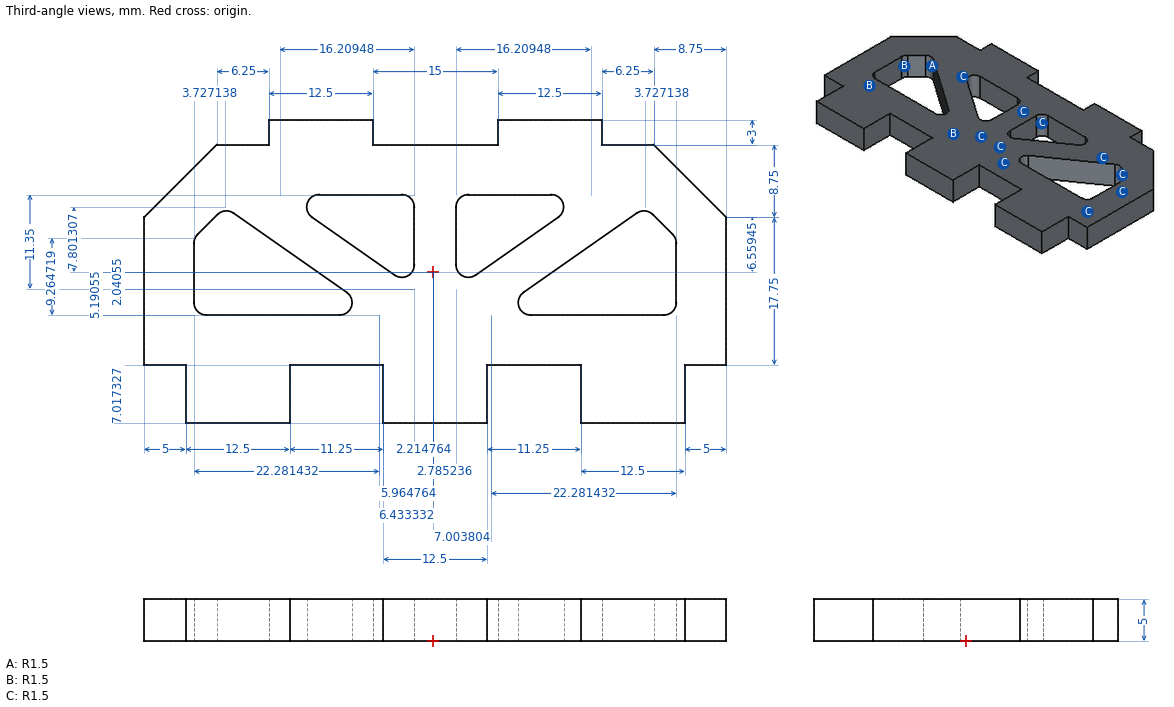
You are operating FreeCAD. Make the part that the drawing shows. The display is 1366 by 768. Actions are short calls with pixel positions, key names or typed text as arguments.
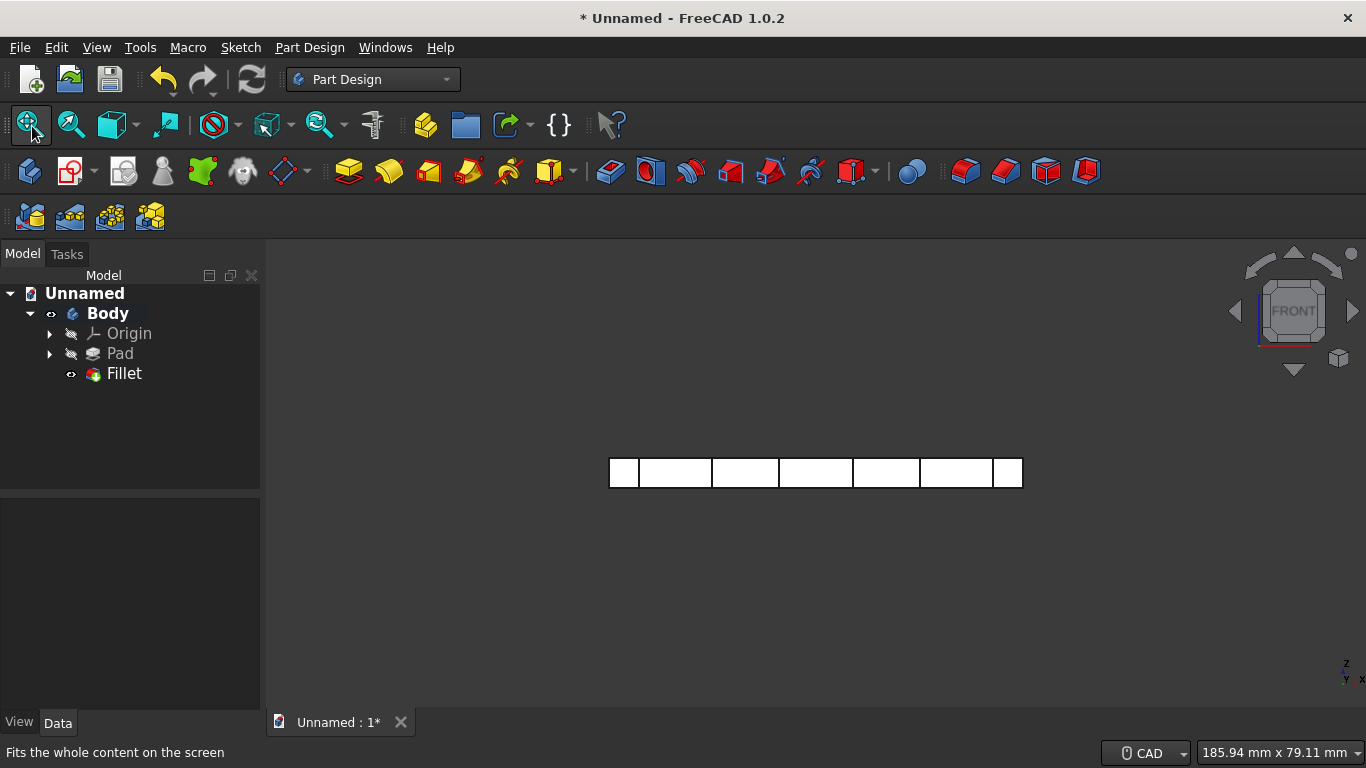
key(3)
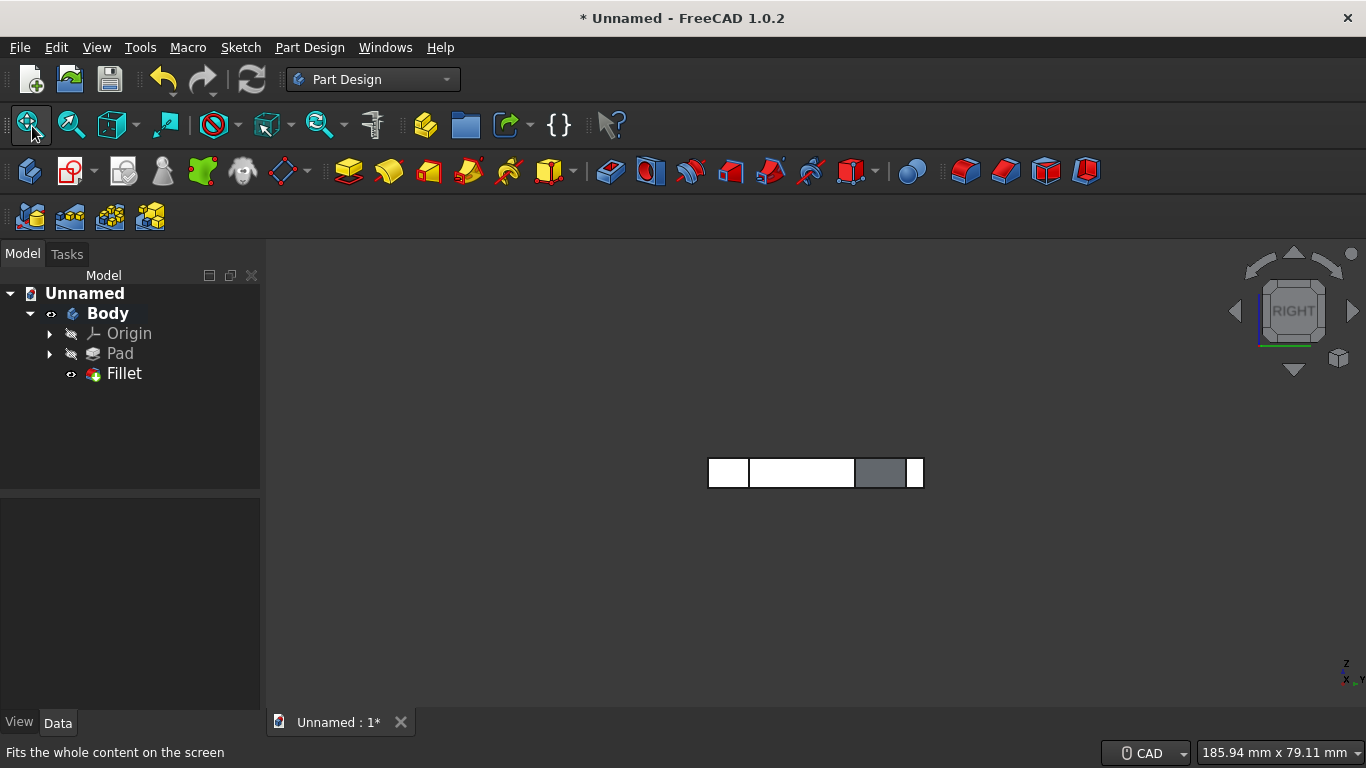
key(v)
key(f)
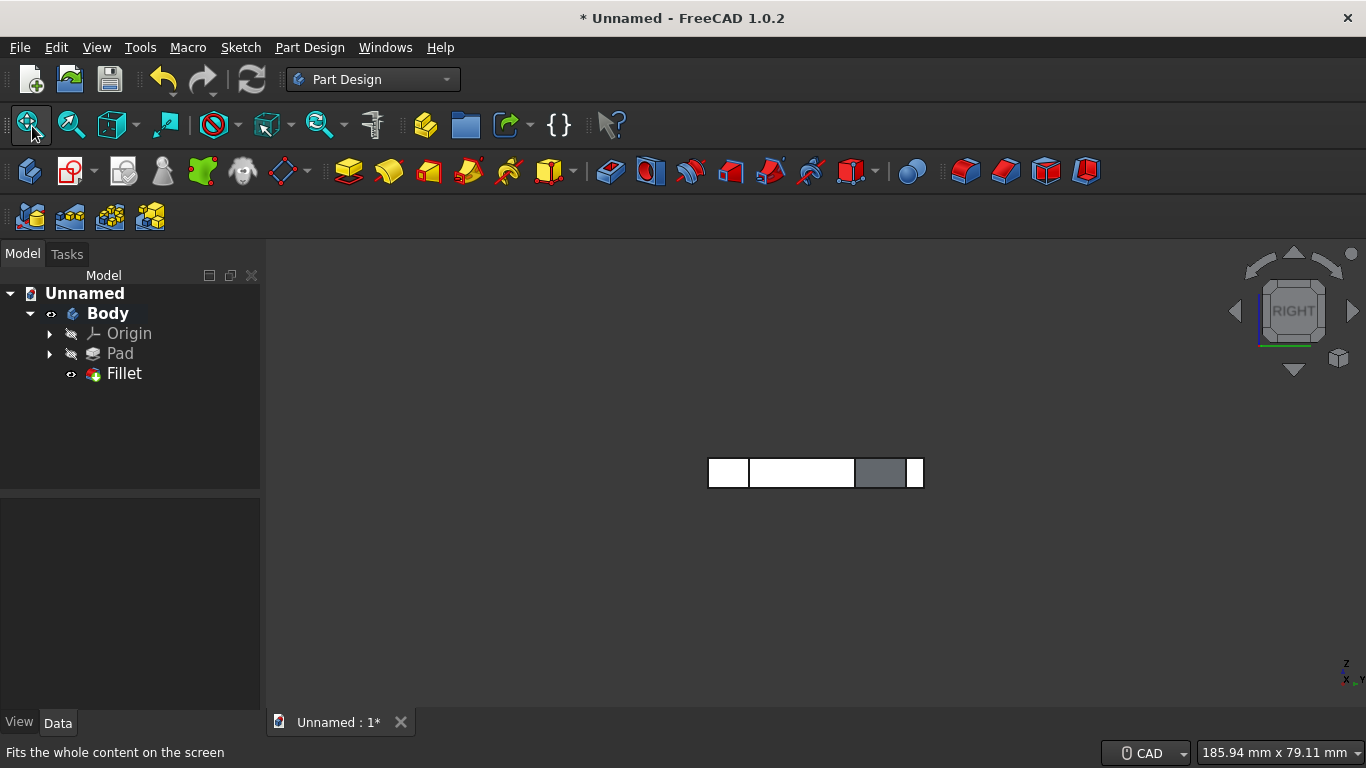
key(5)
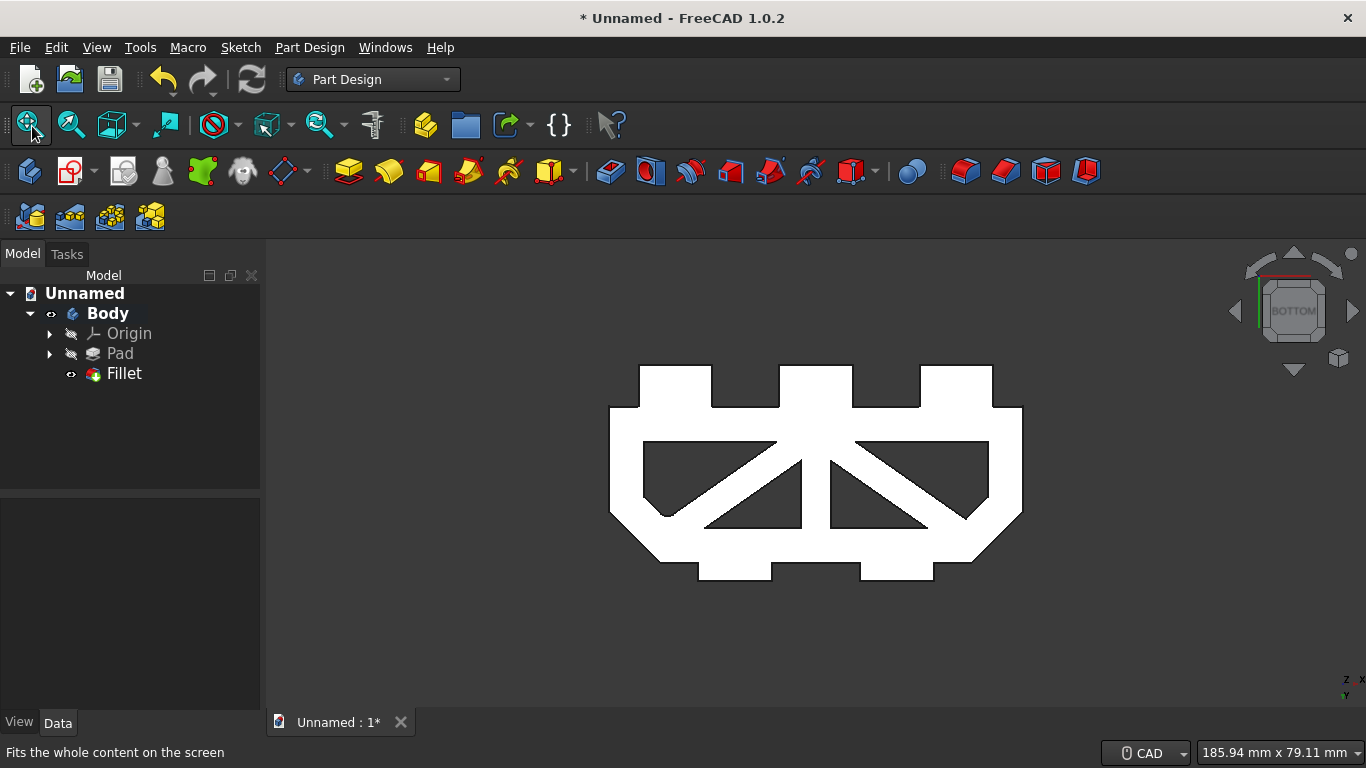
key(4)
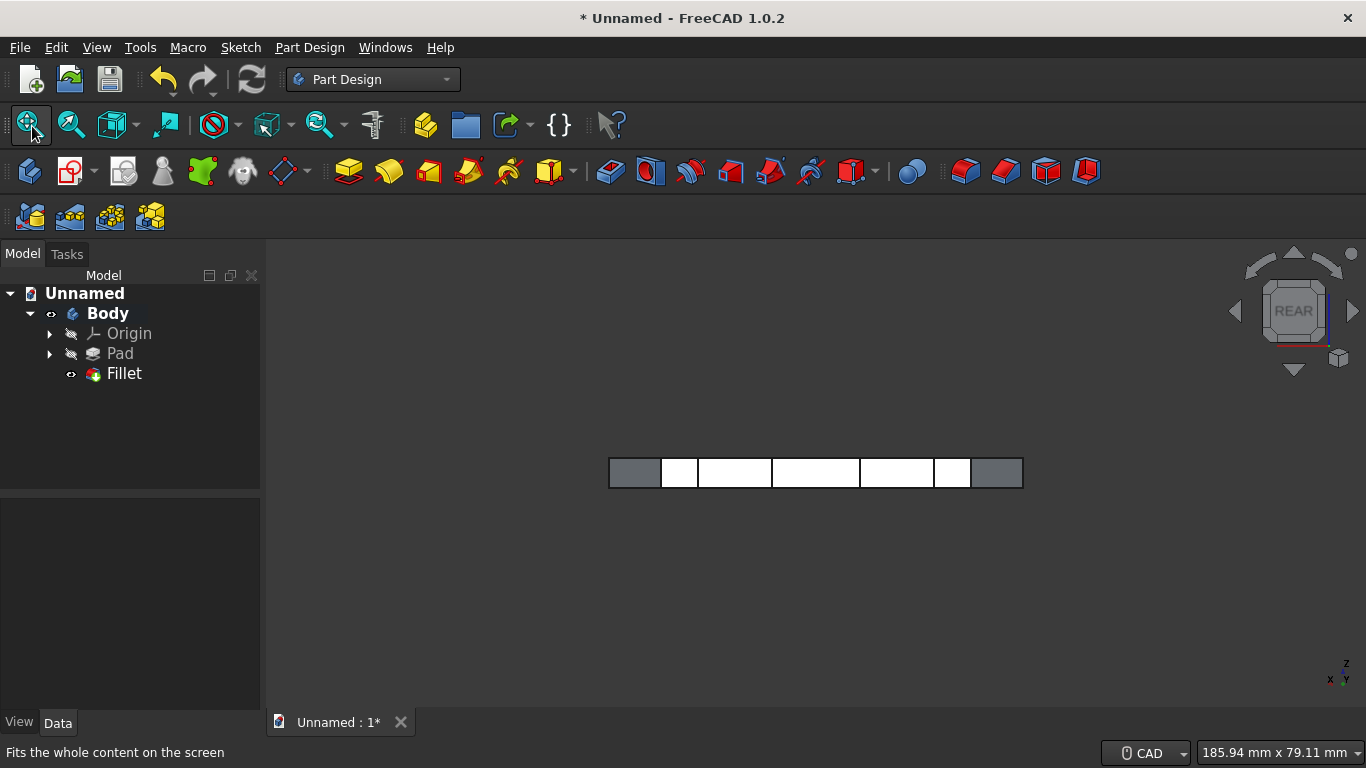
key(v)
key(f)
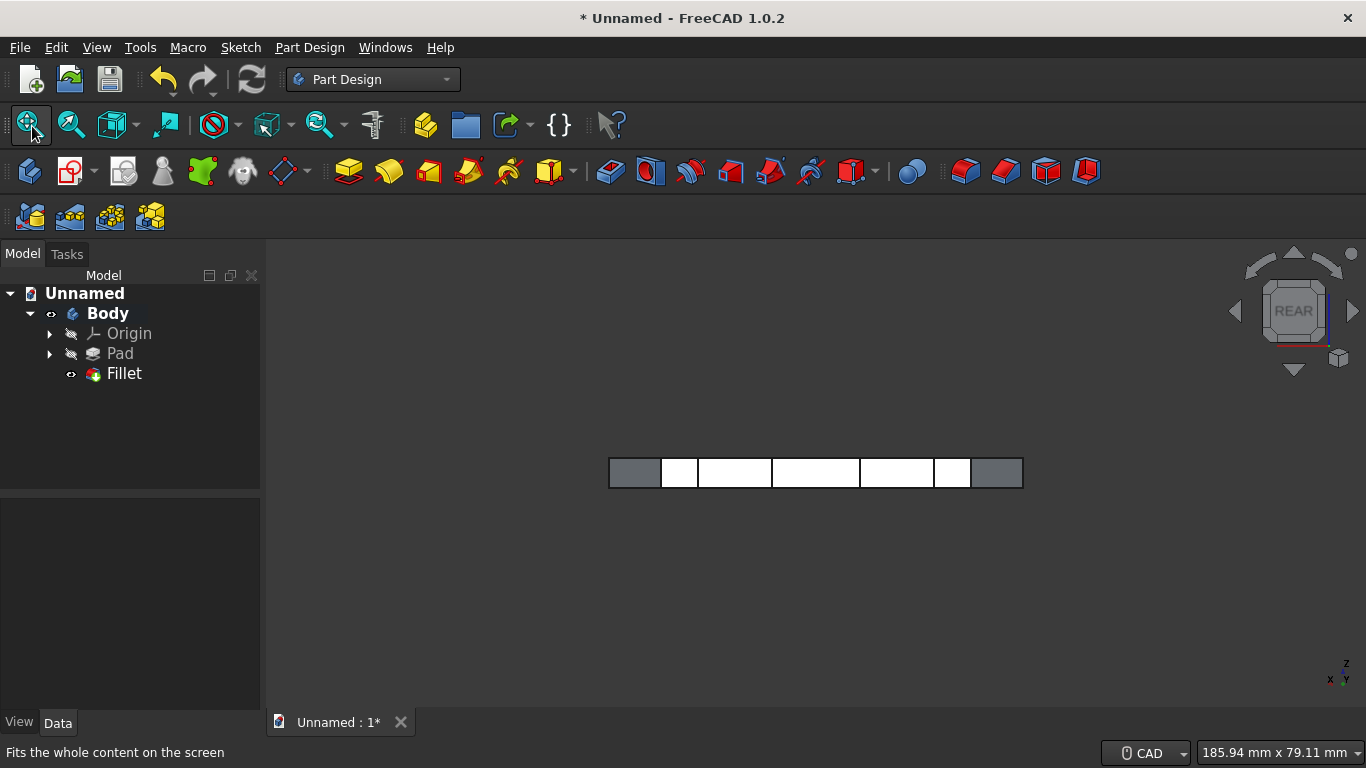
key(6)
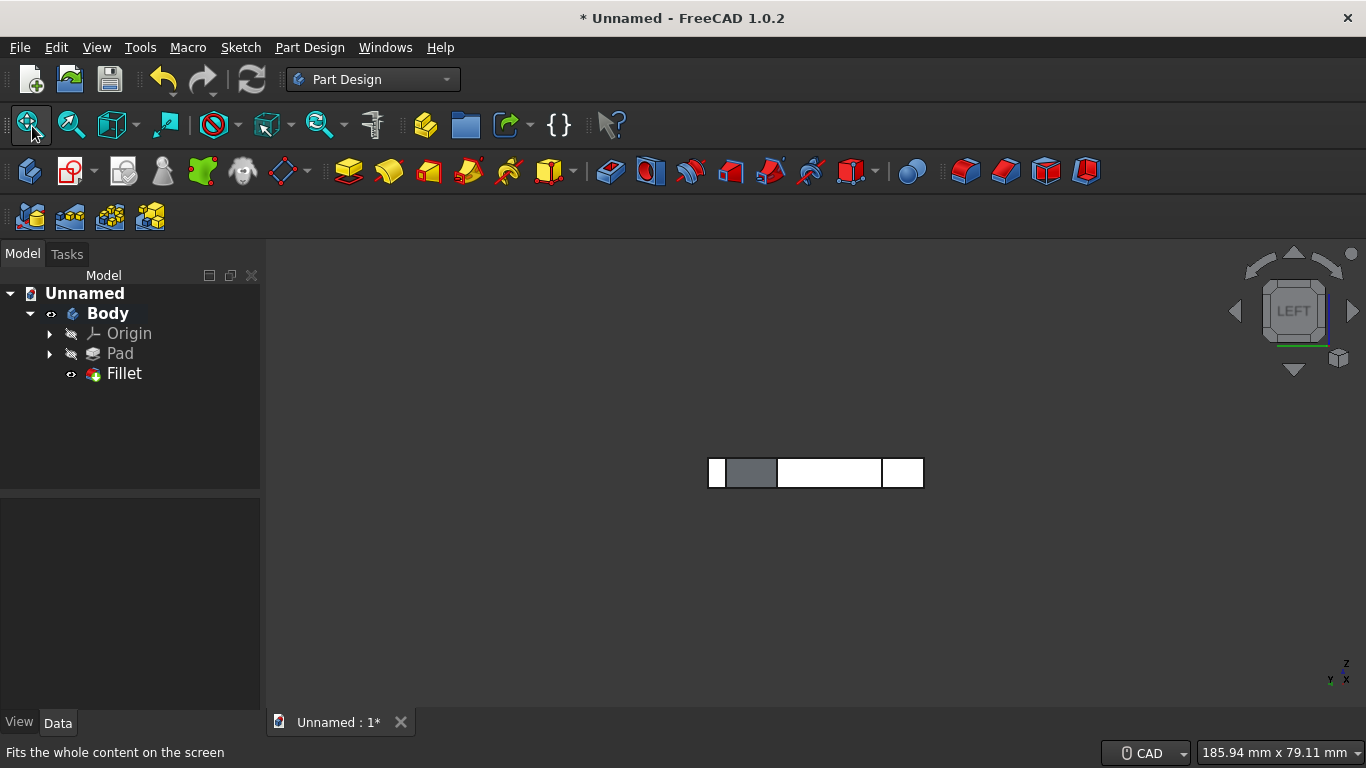
key(v)
key(f)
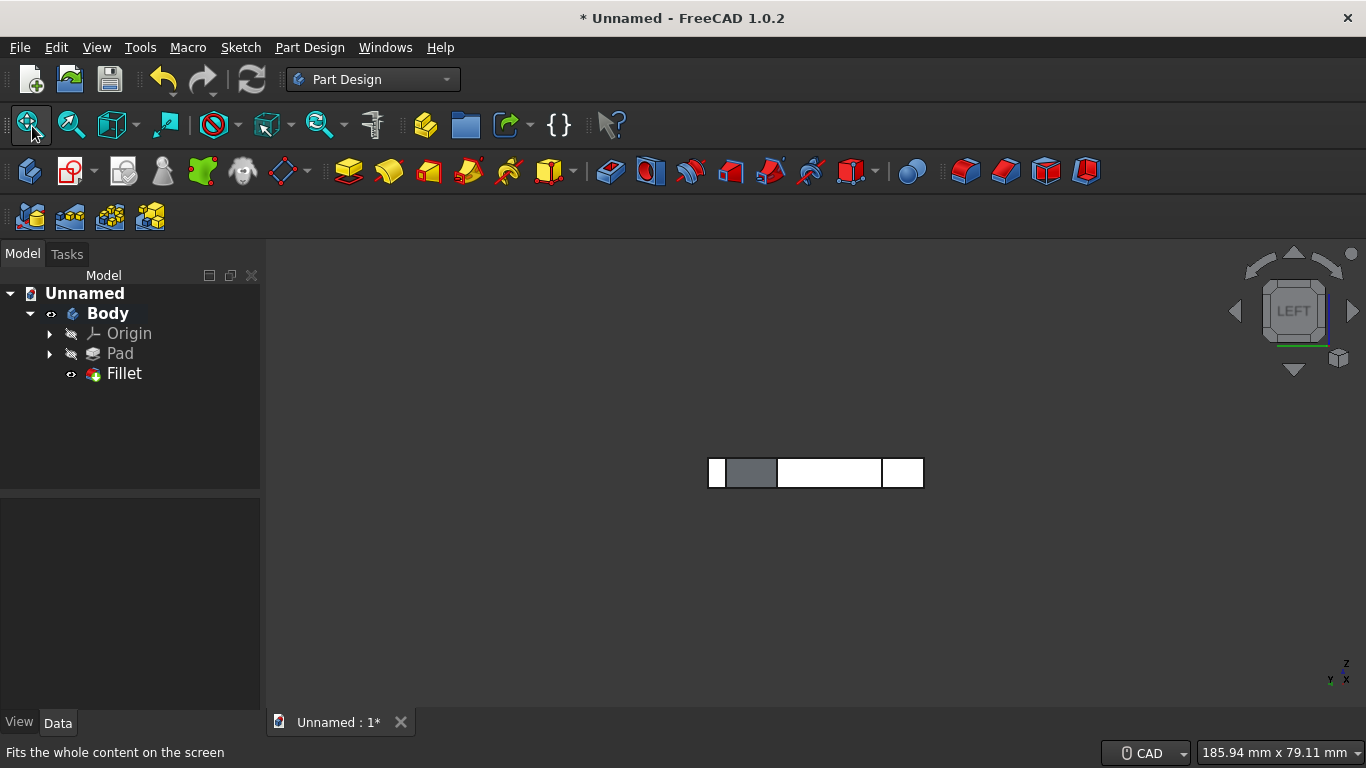
key(v)
key(3)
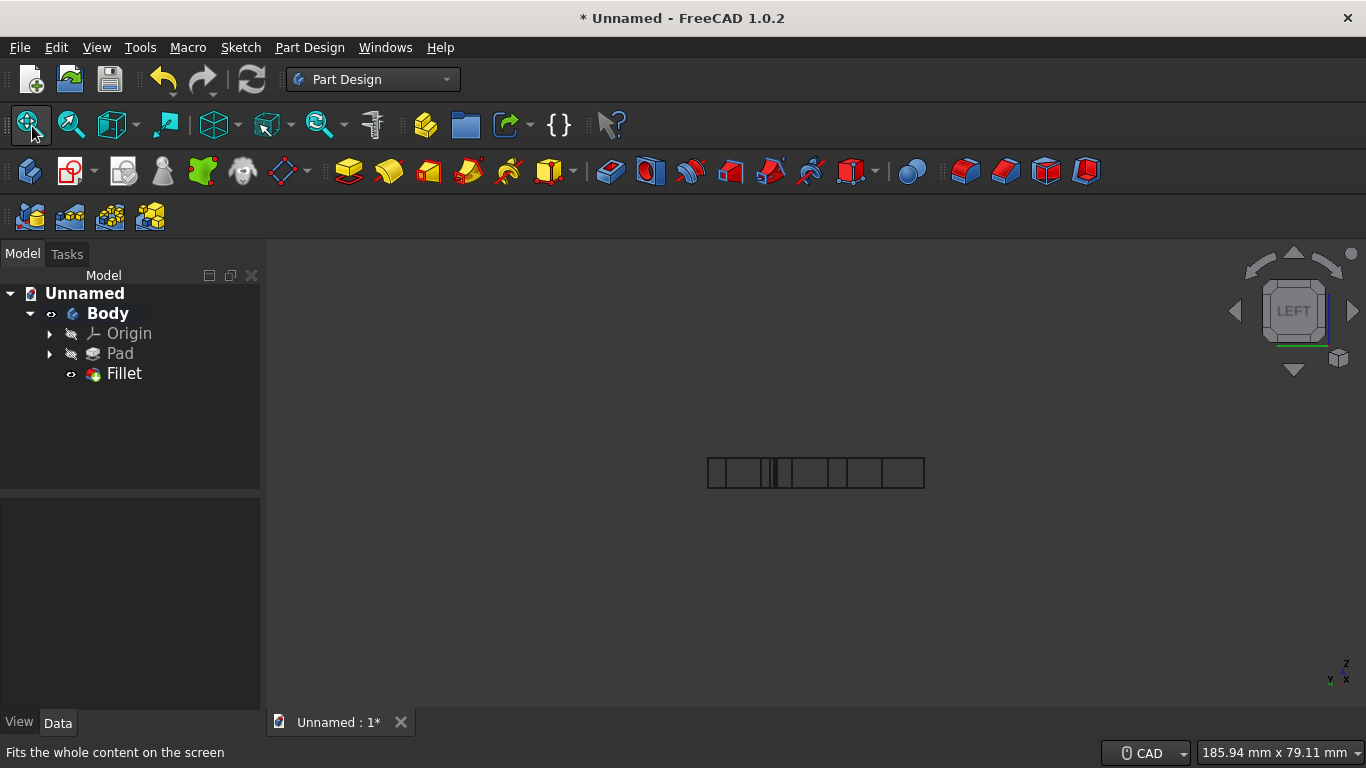
key(0)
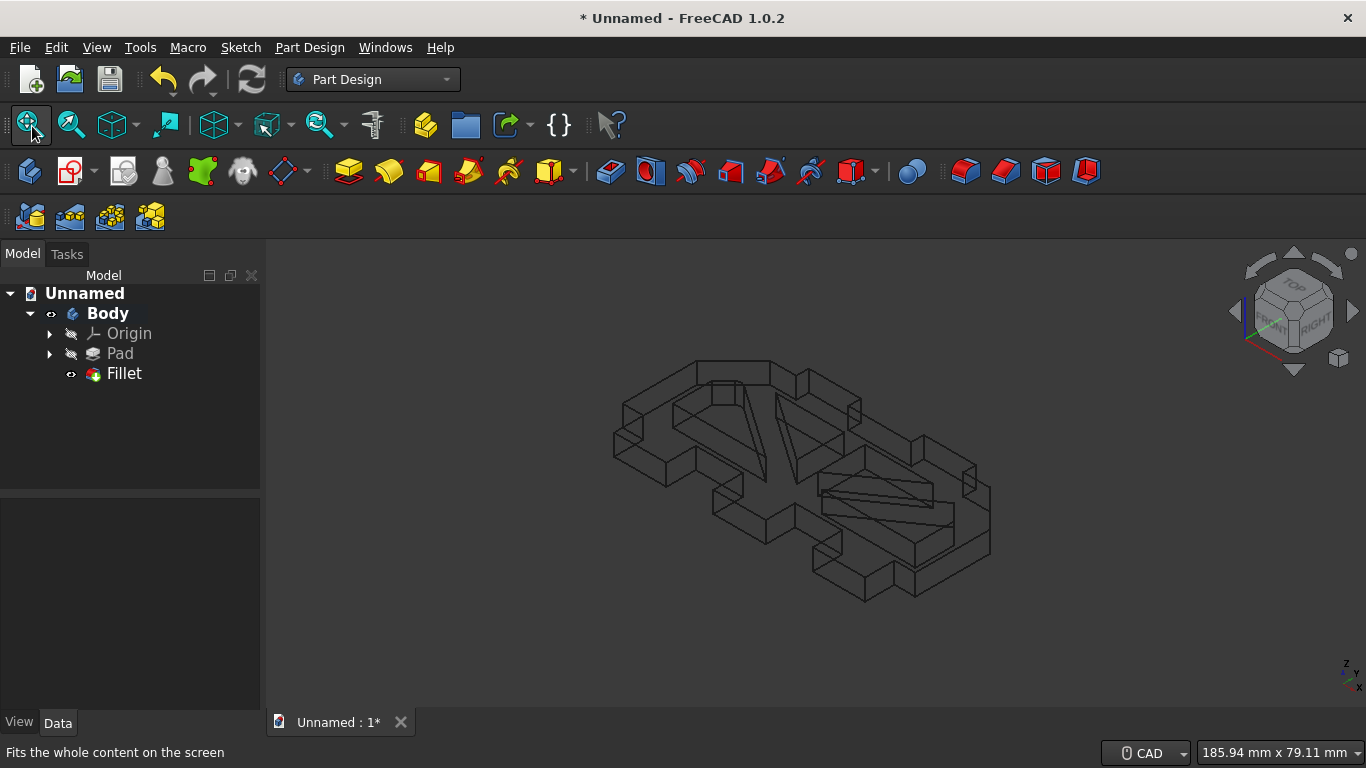
click(766, 468)